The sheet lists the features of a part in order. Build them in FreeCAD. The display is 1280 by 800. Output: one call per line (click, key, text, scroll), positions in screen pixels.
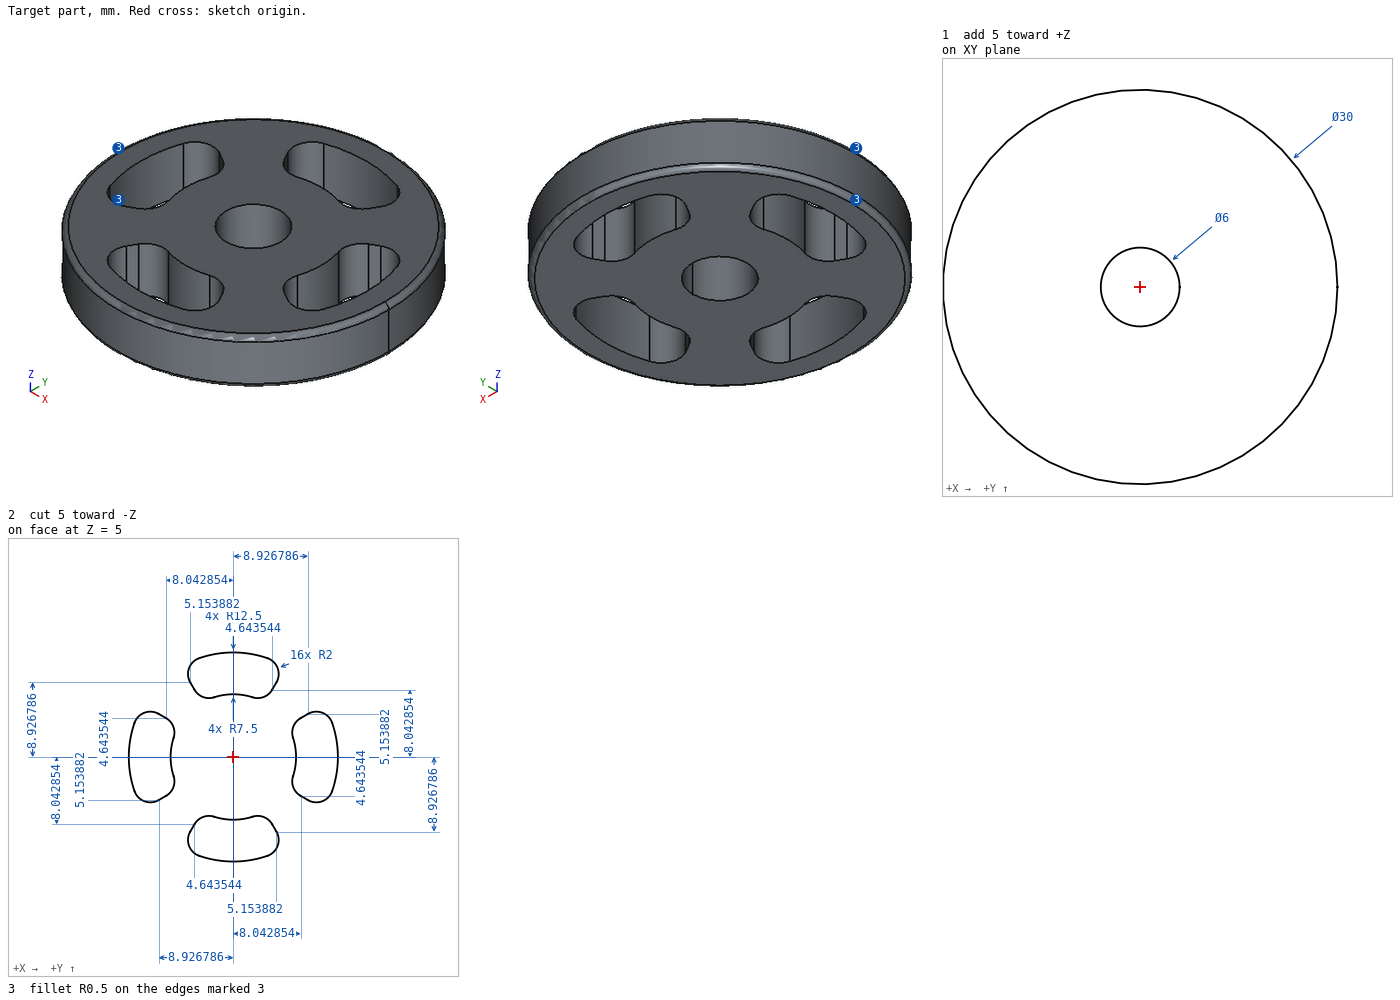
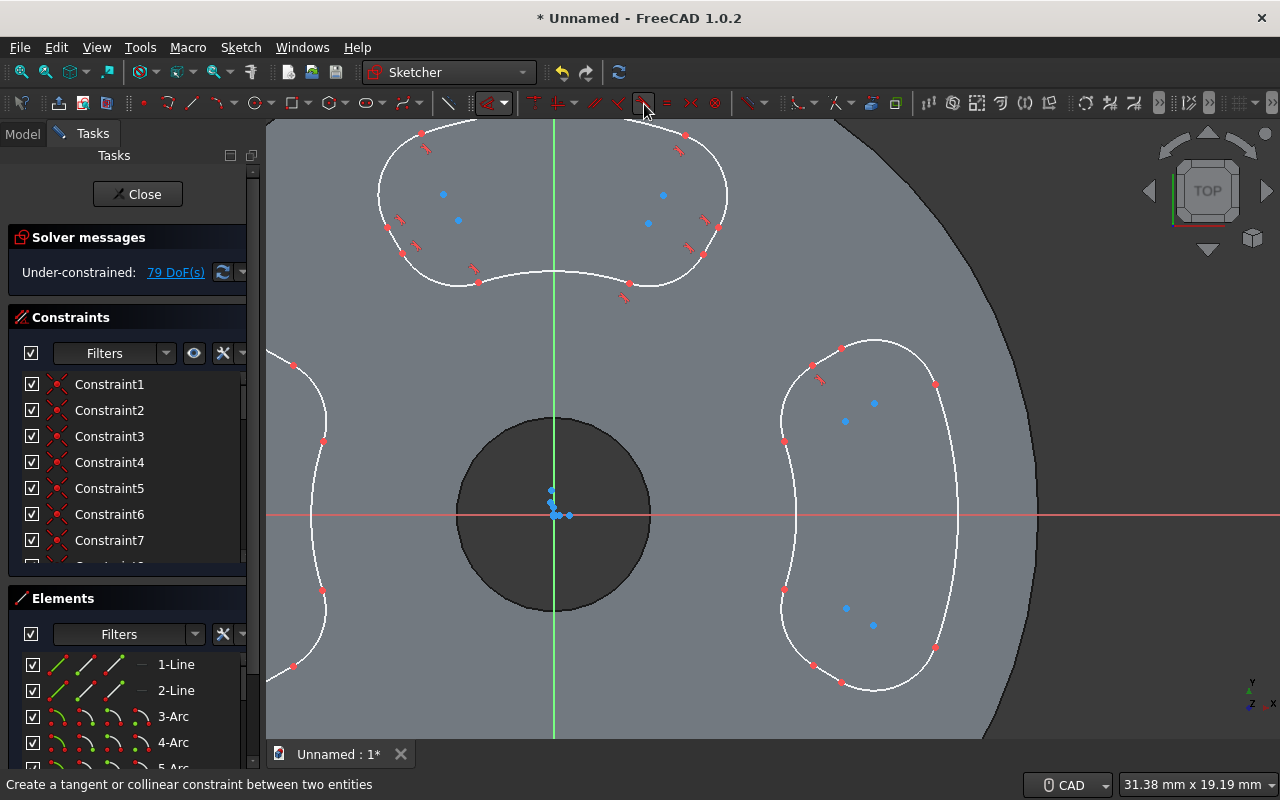
scroll(833, 354, up, 2)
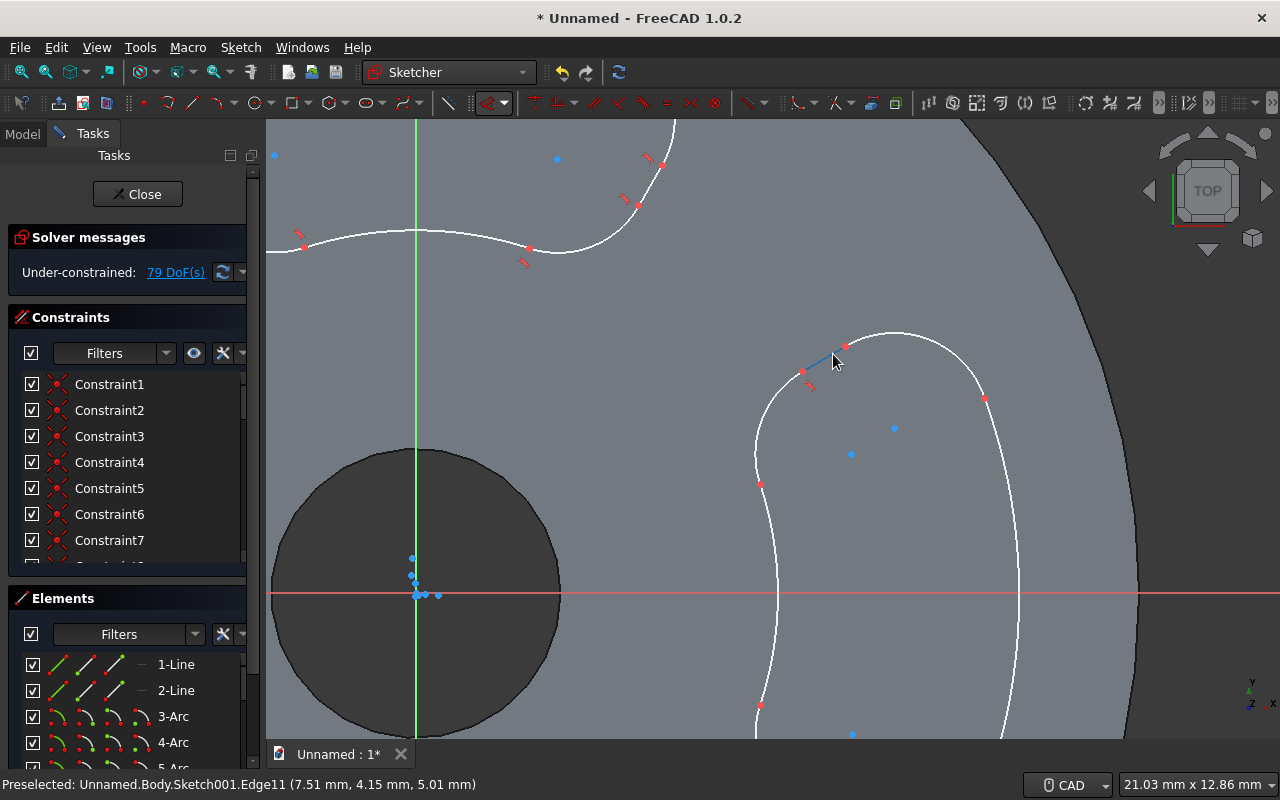
click(833, 354)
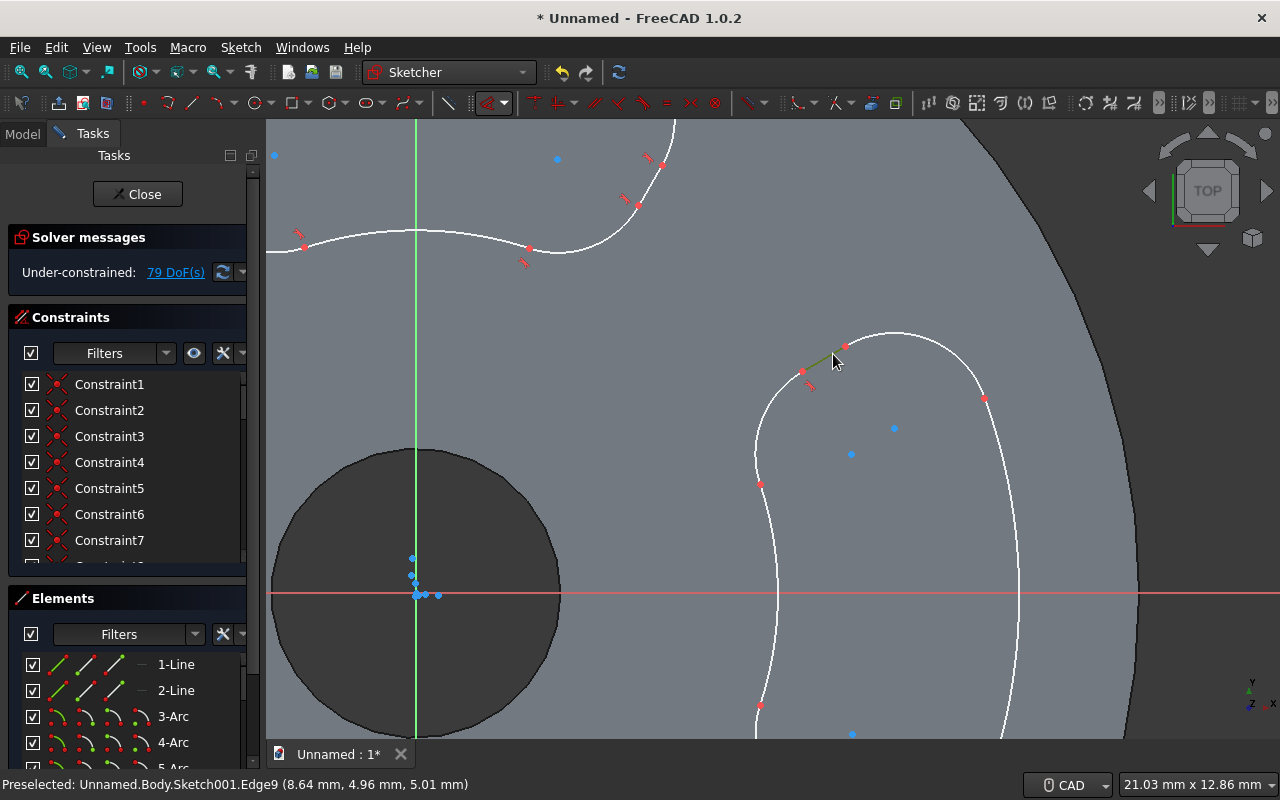
click(957, 357)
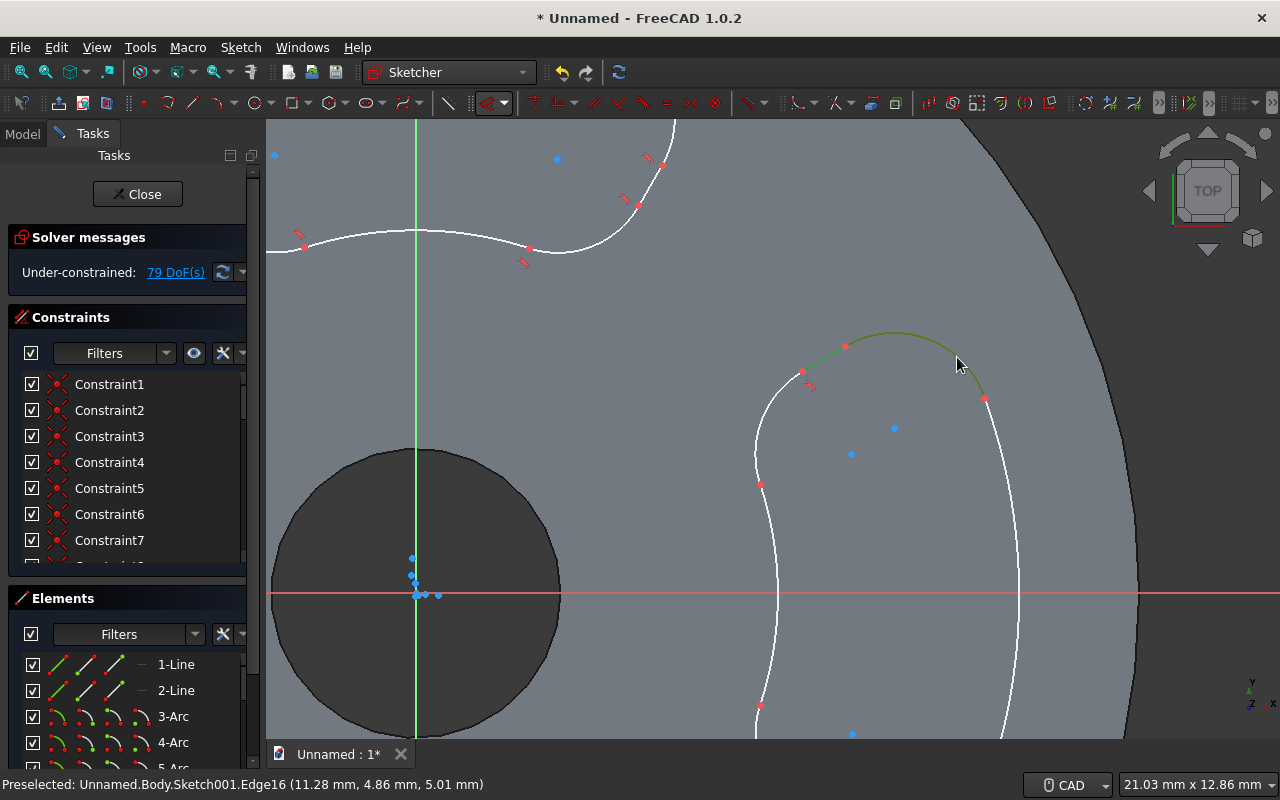
click(644, 104)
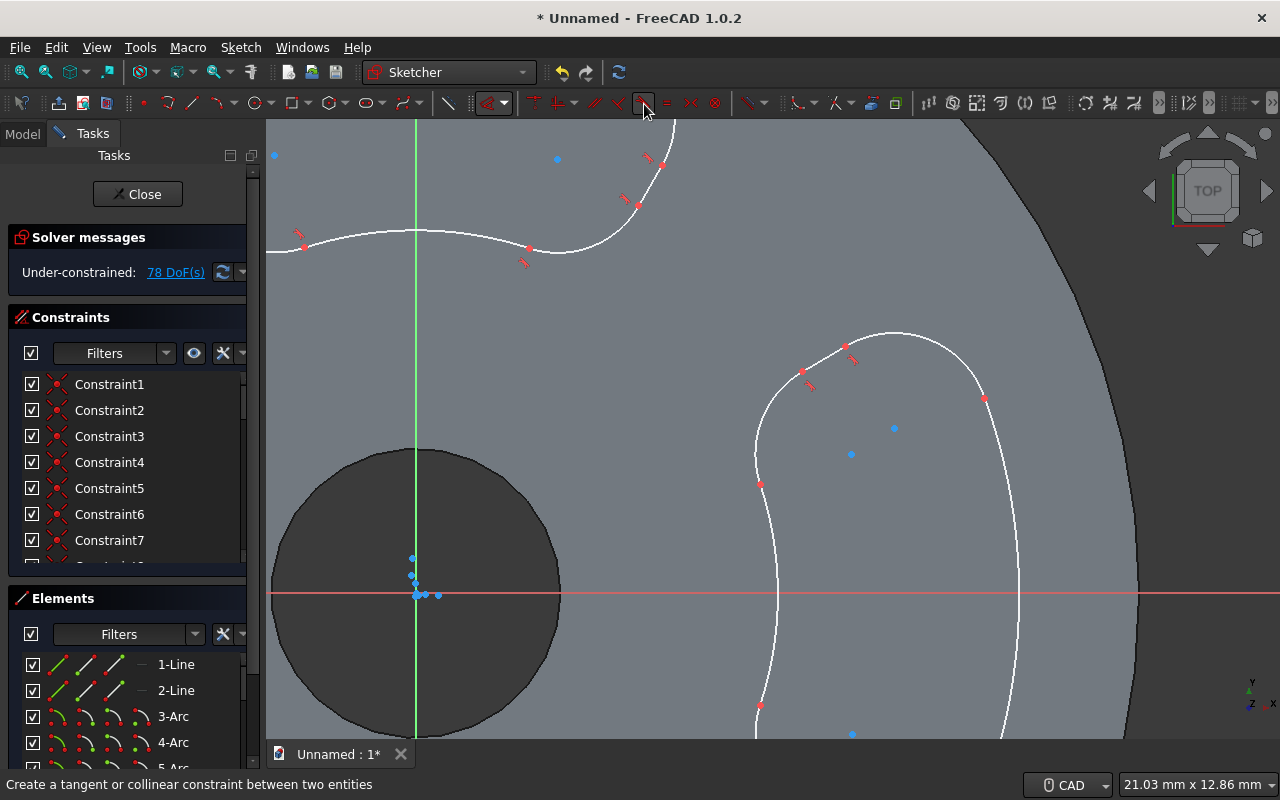
scroll(829, 358, down, 6)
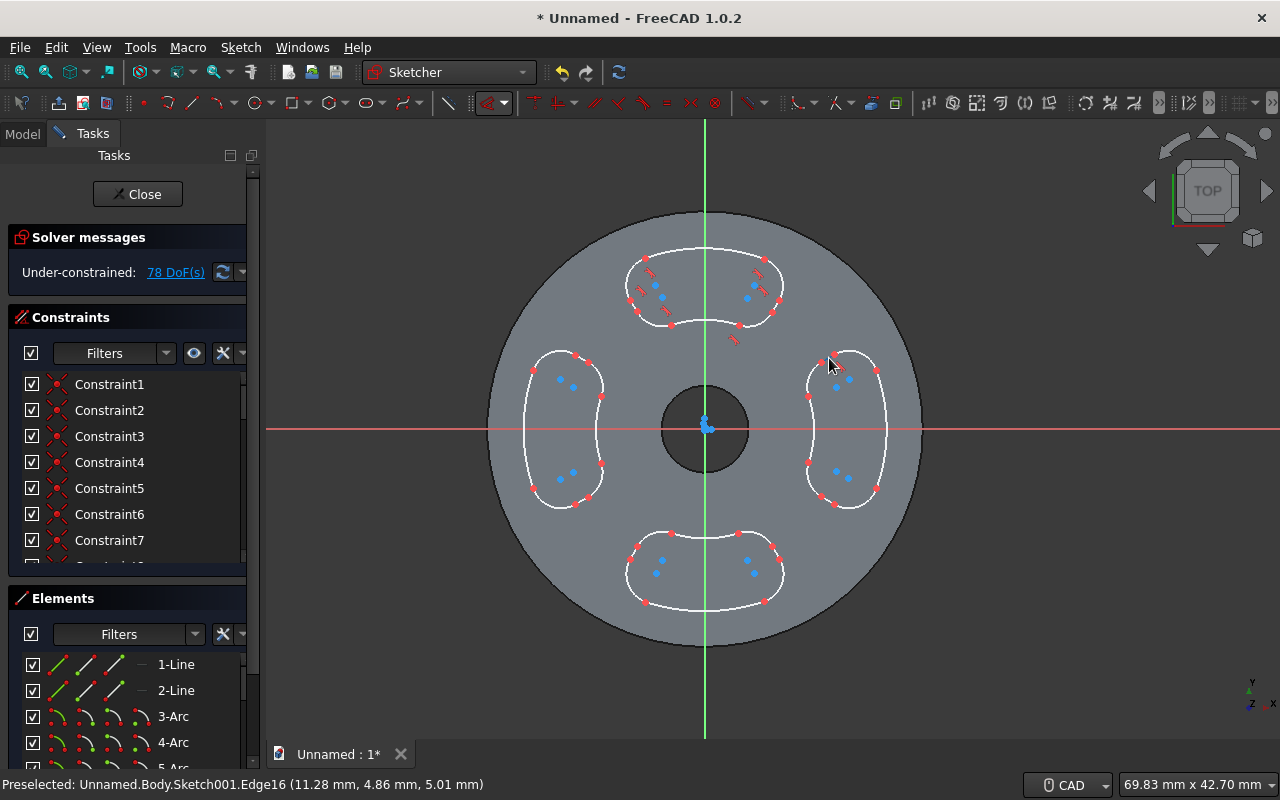
scroll(826, 499, up, 6)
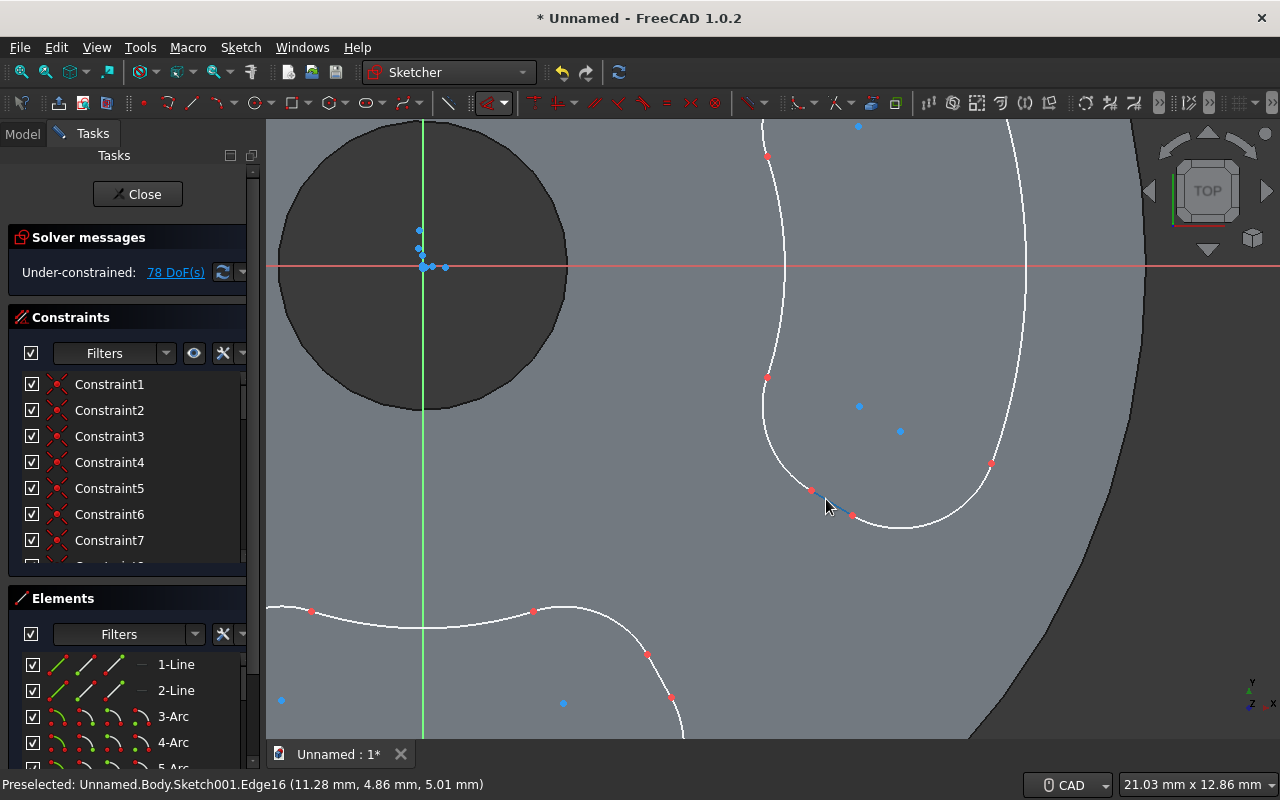
click(824, 498)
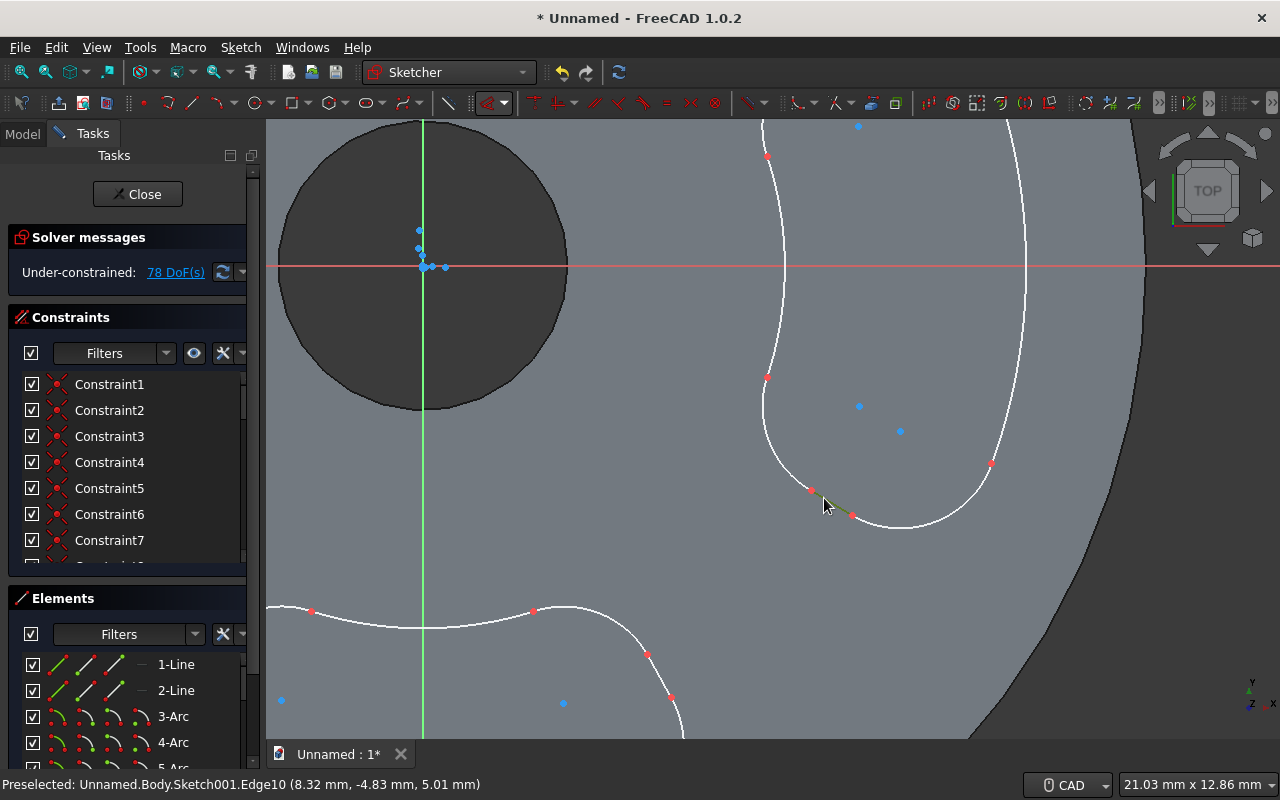
click(763, 416)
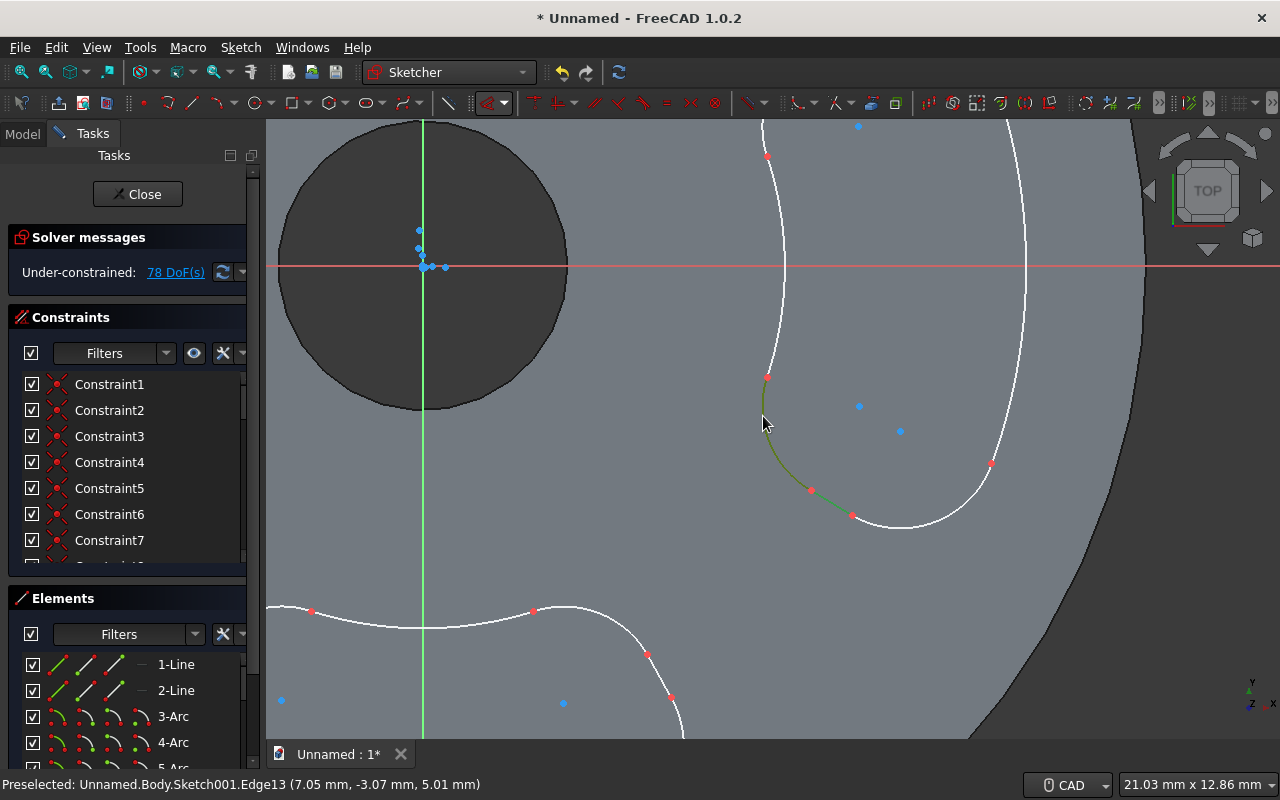
click(644, 104)